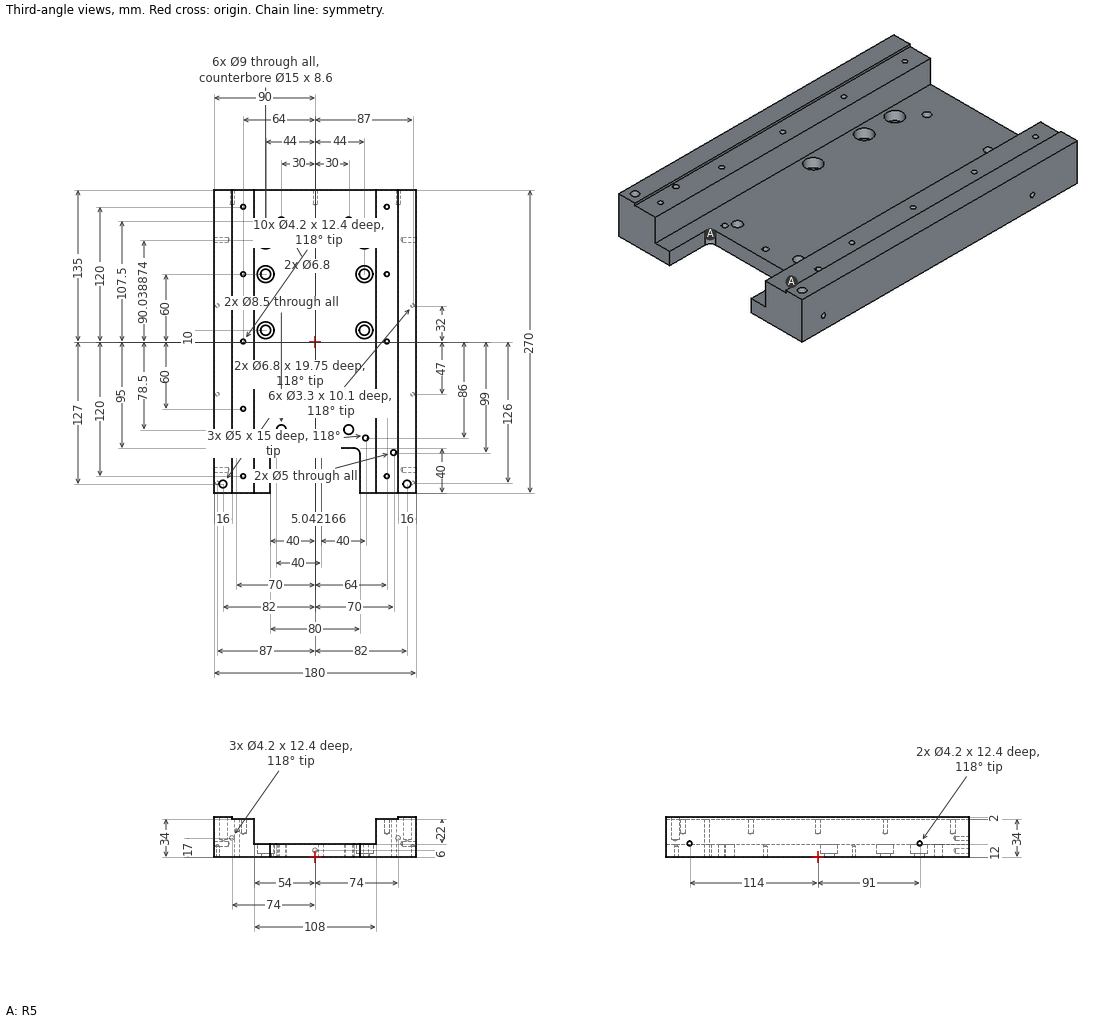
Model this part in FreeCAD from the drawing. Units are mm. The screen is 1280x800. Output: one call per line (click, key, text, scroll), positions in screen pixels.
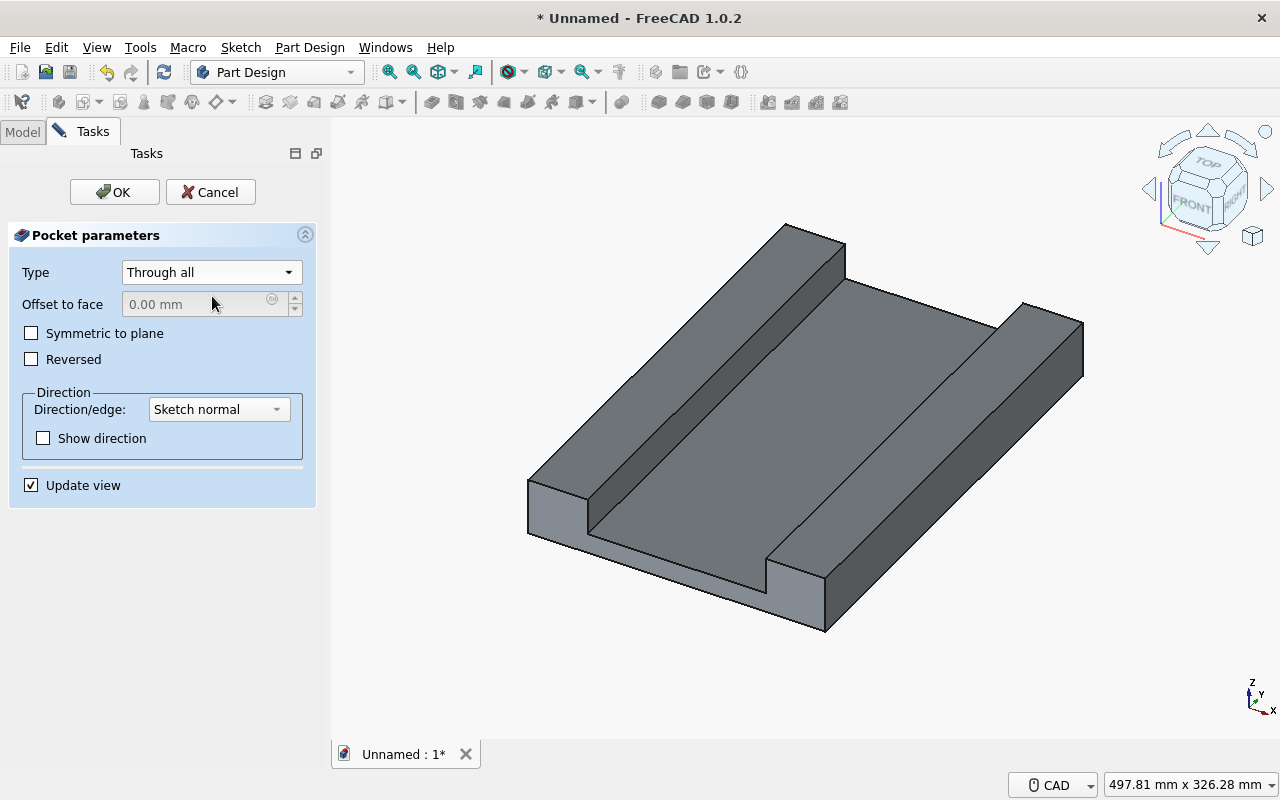
click(115, 192)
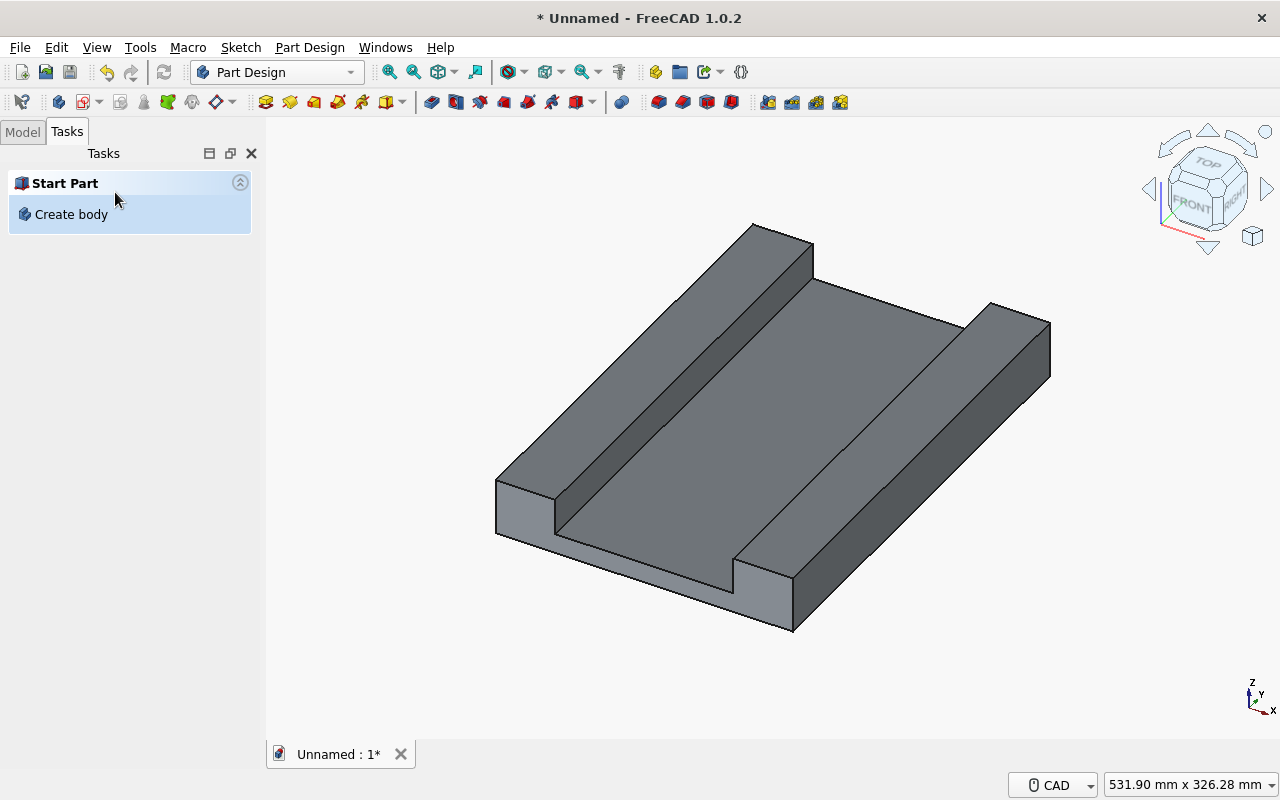
click(764, 252)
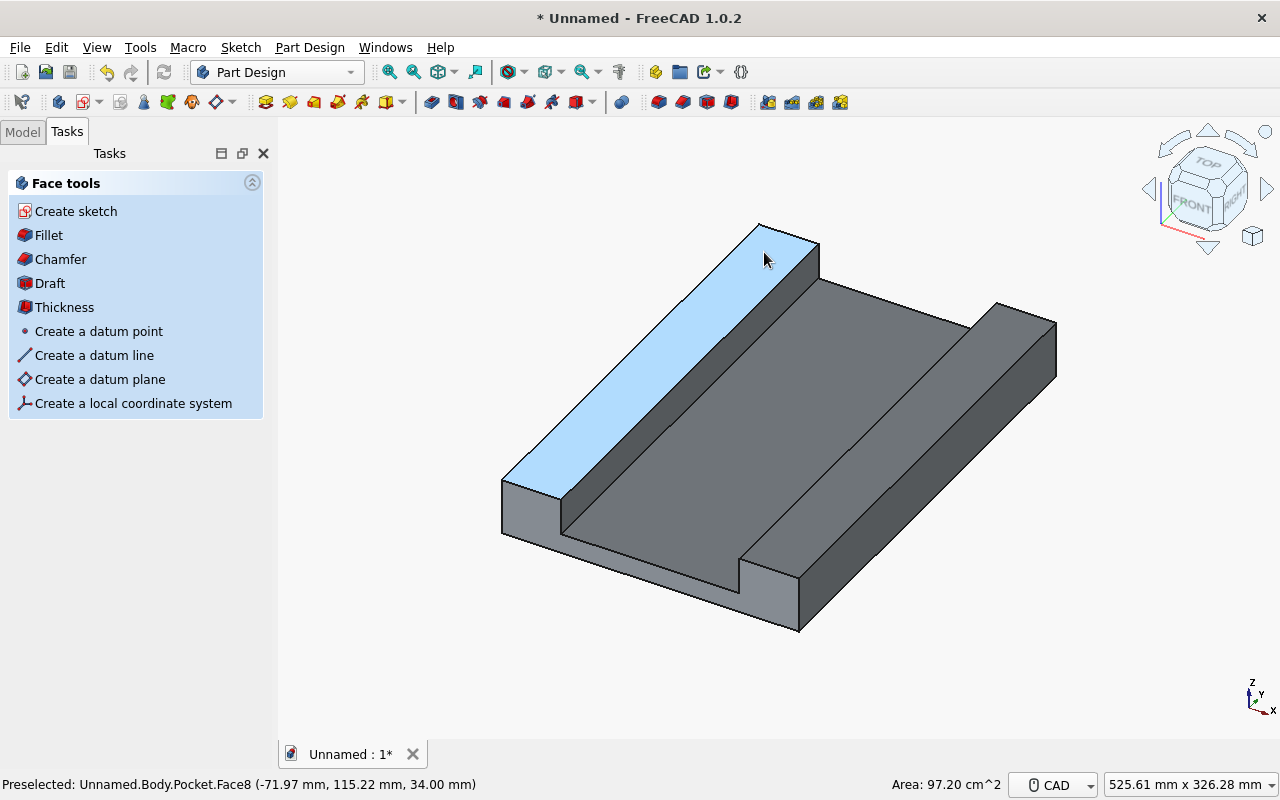
click(84, 102)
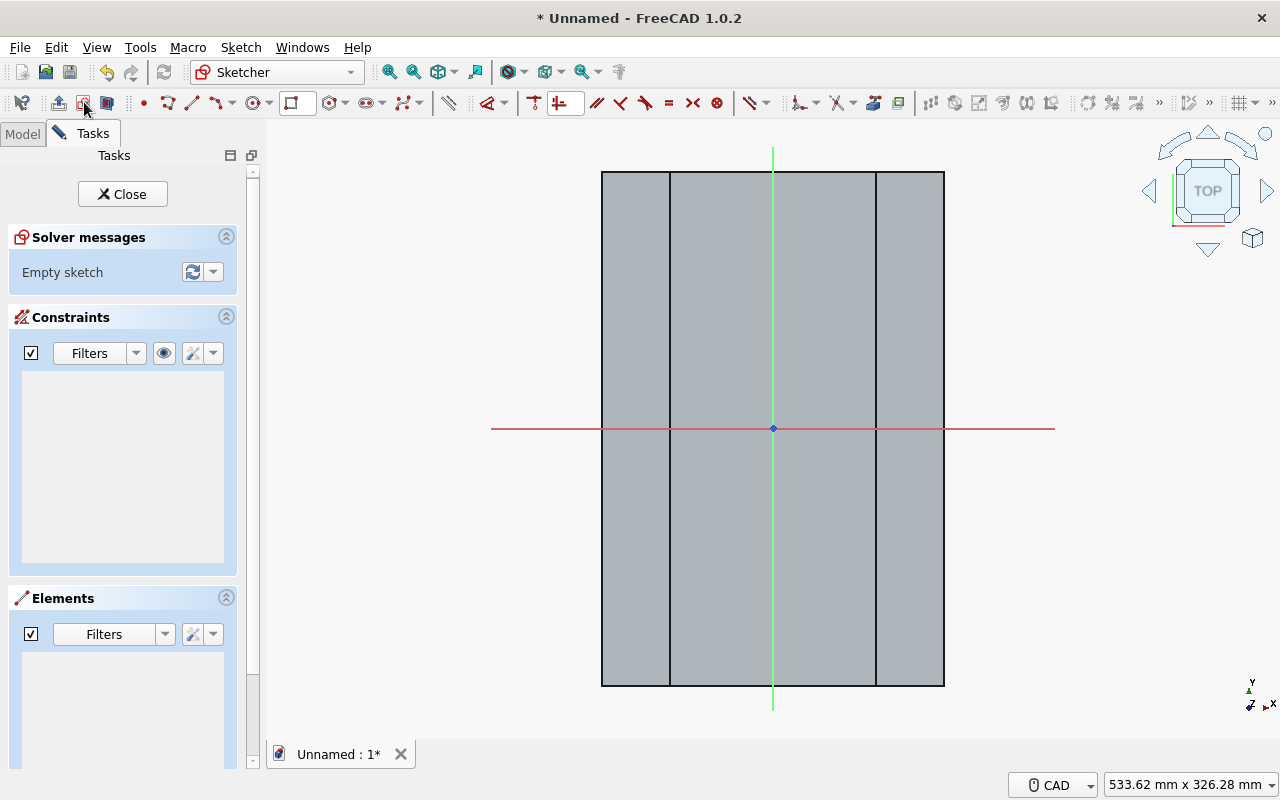
click(292, 104)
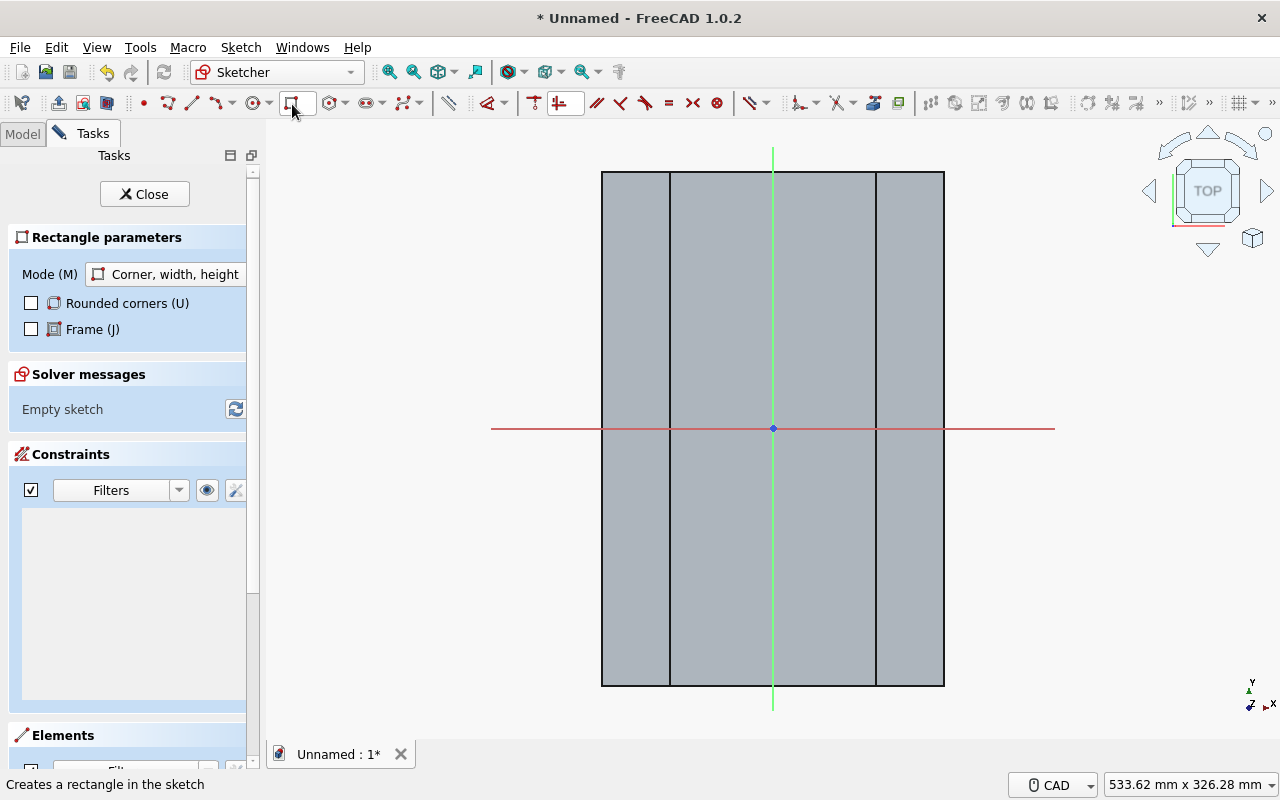
click(602, 172)
move(632, 686)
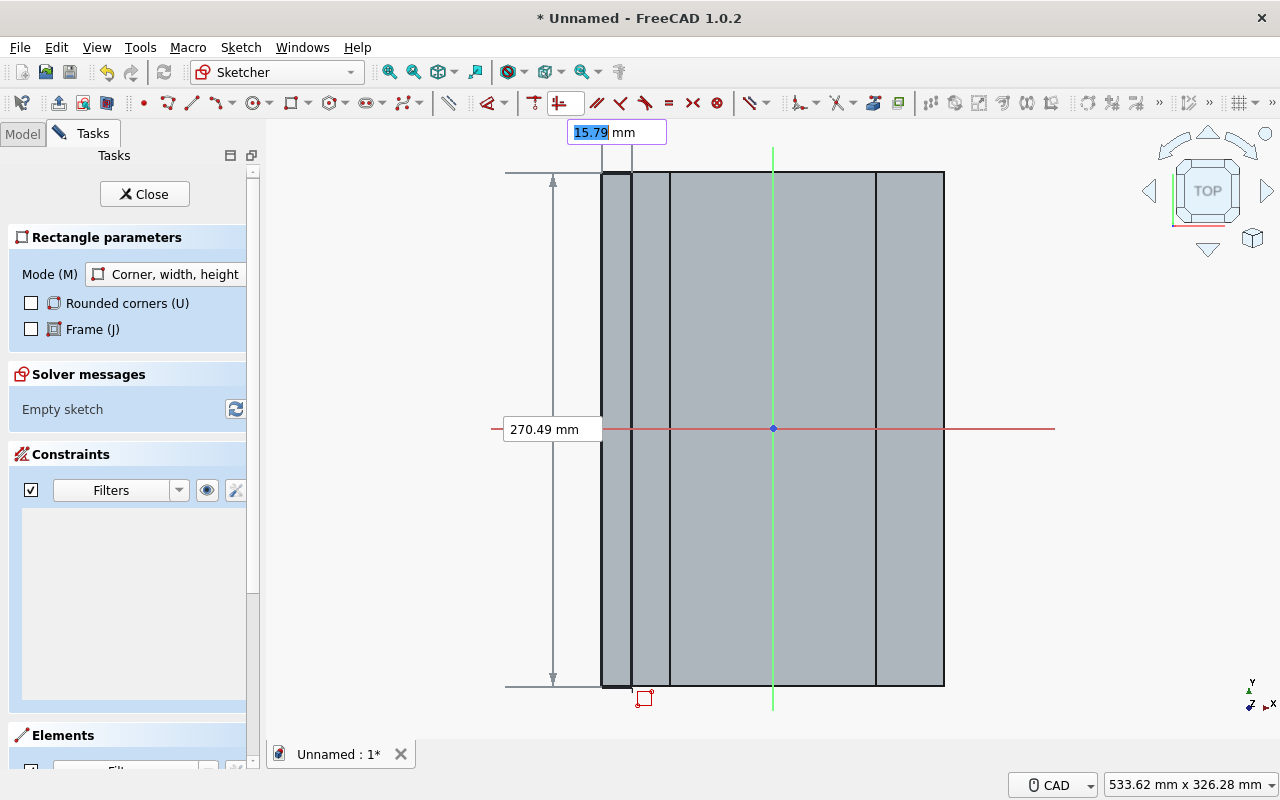
text(16)
key(Tab)
text(270)
key(Return)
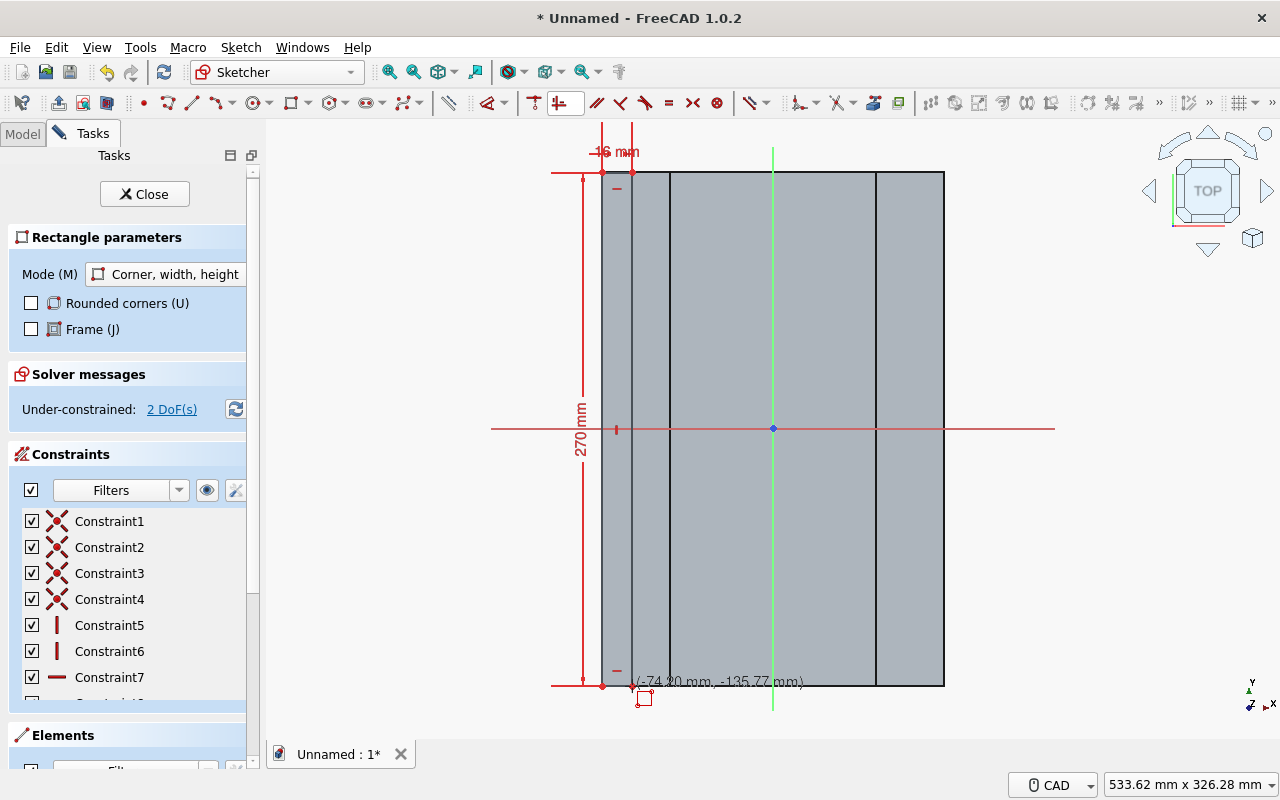
click(914, 172)
move(944, 686)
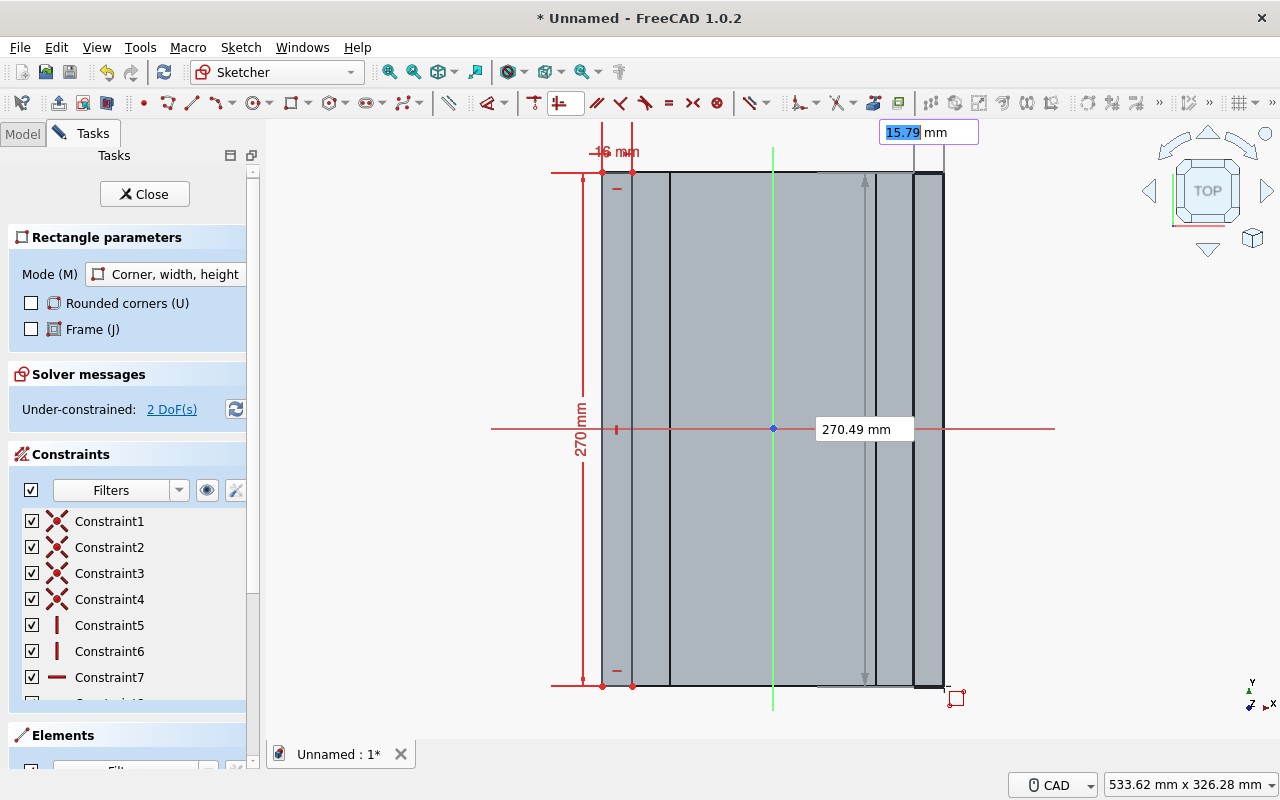
text(16)
key(Tab)
text(270)
key(Return)
key(Escape)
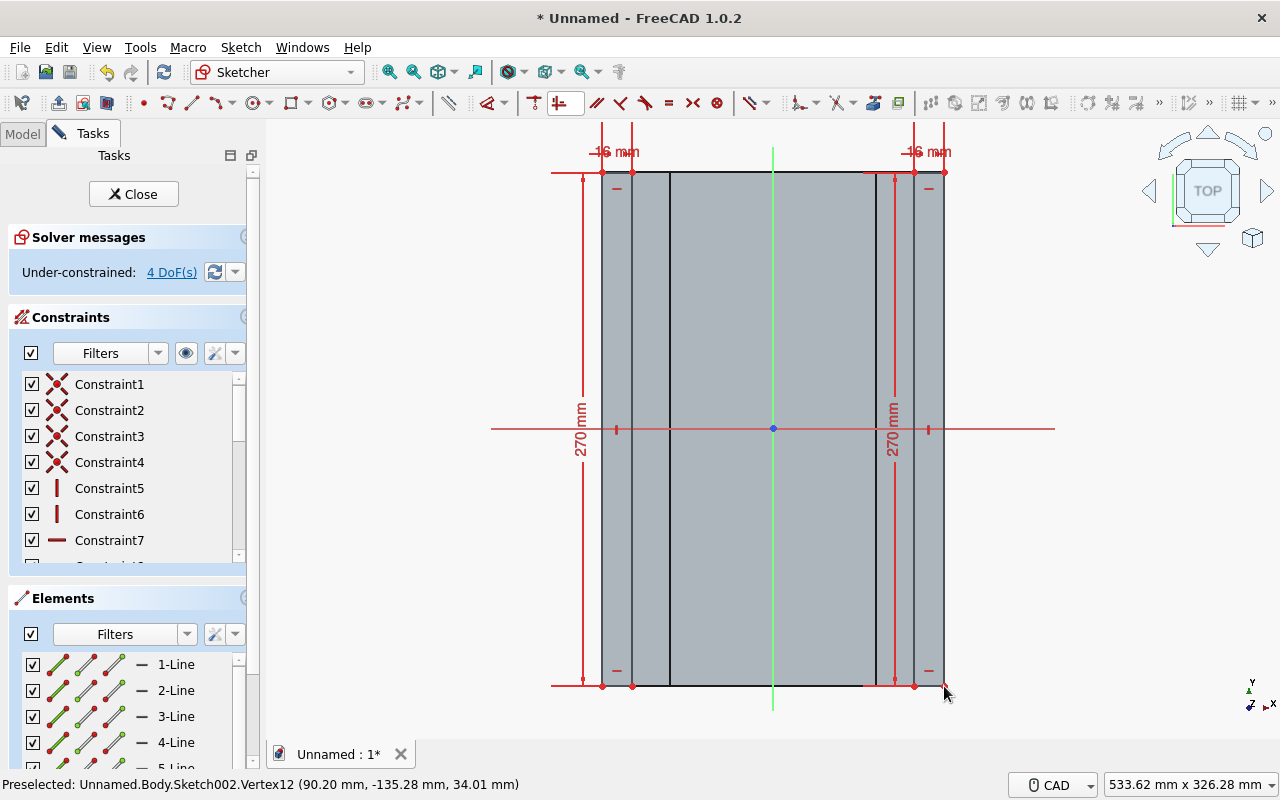
click(632, 173)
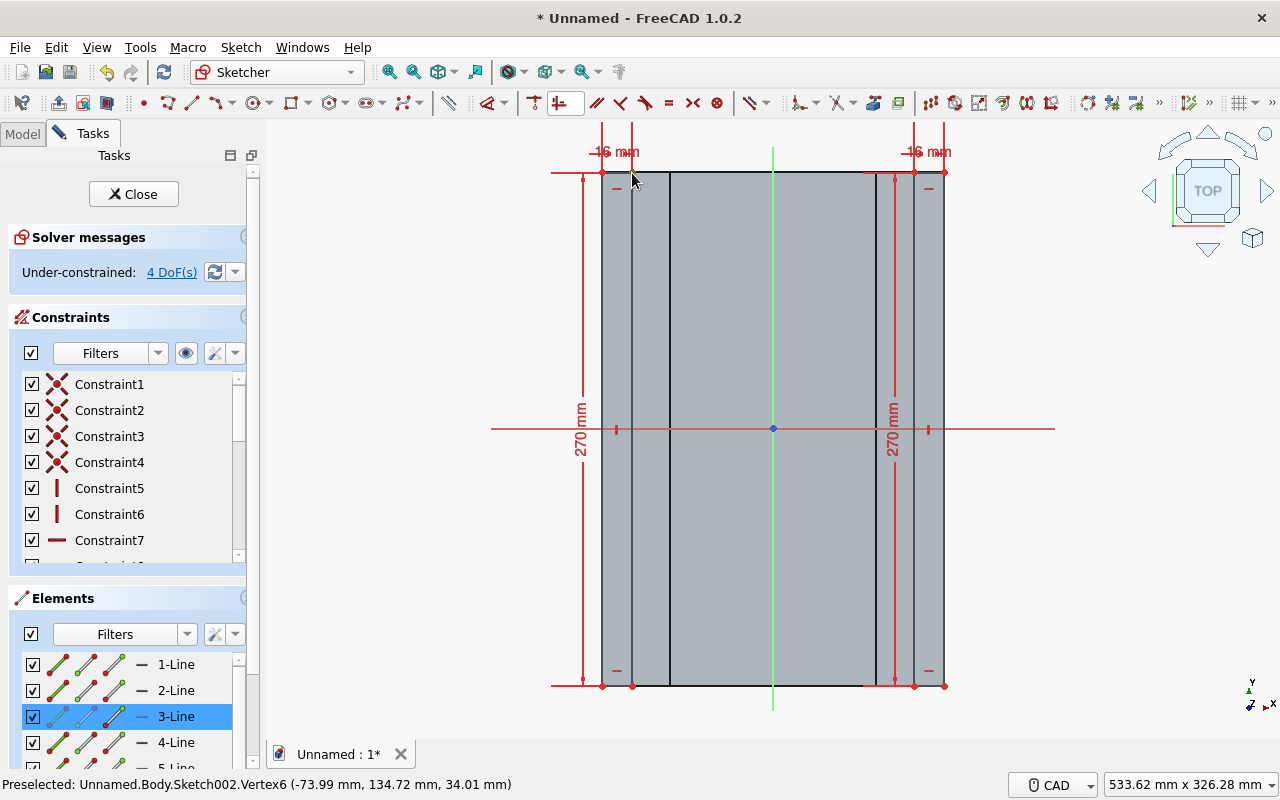
click(914, 173)